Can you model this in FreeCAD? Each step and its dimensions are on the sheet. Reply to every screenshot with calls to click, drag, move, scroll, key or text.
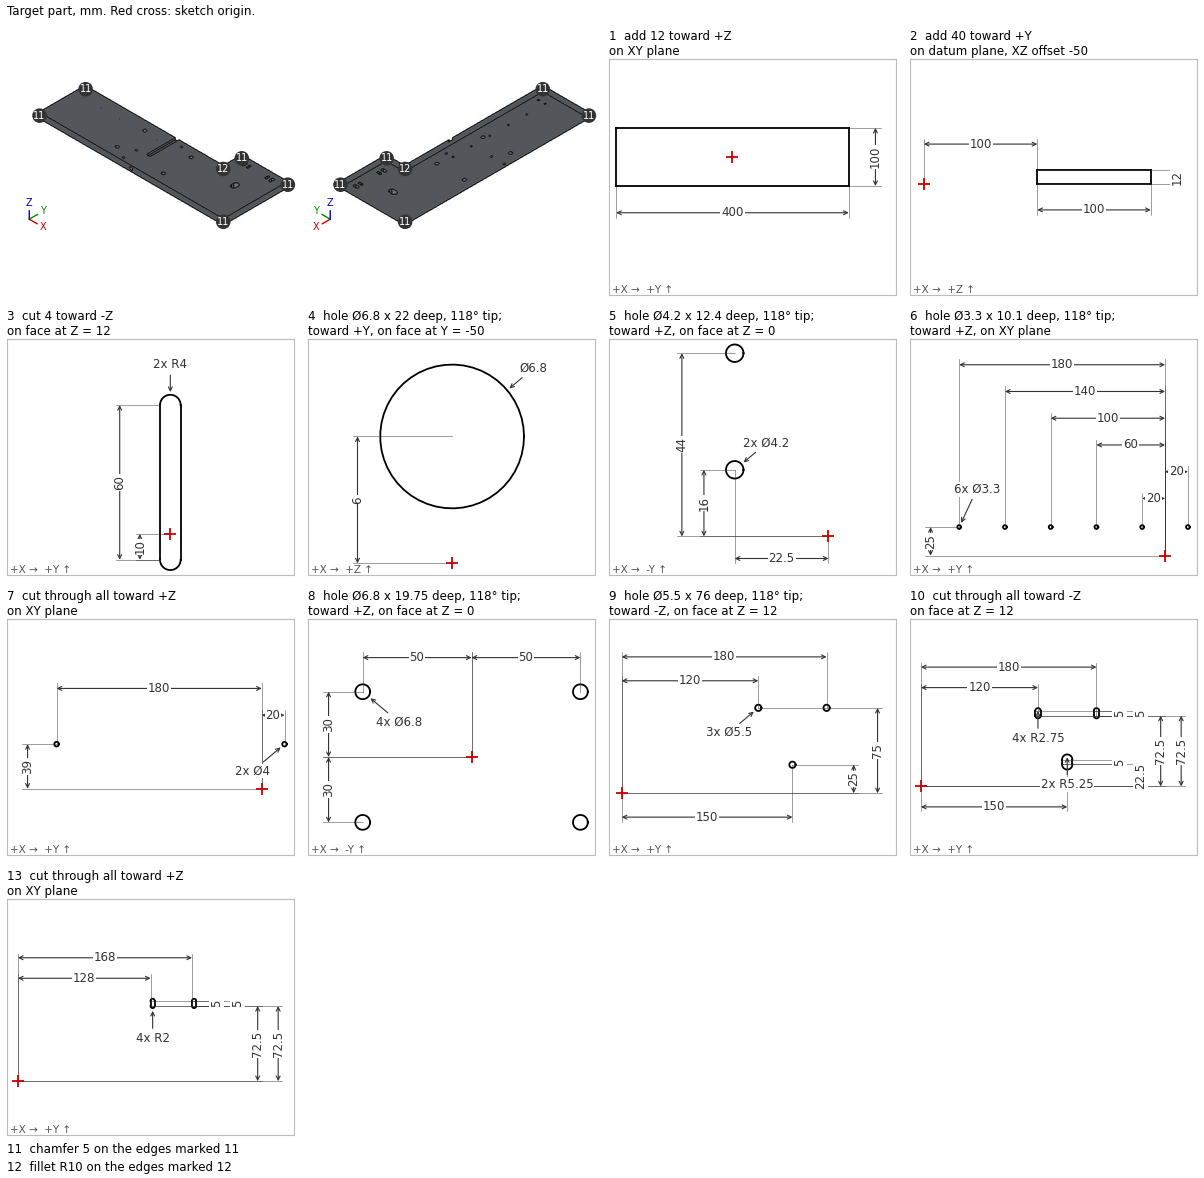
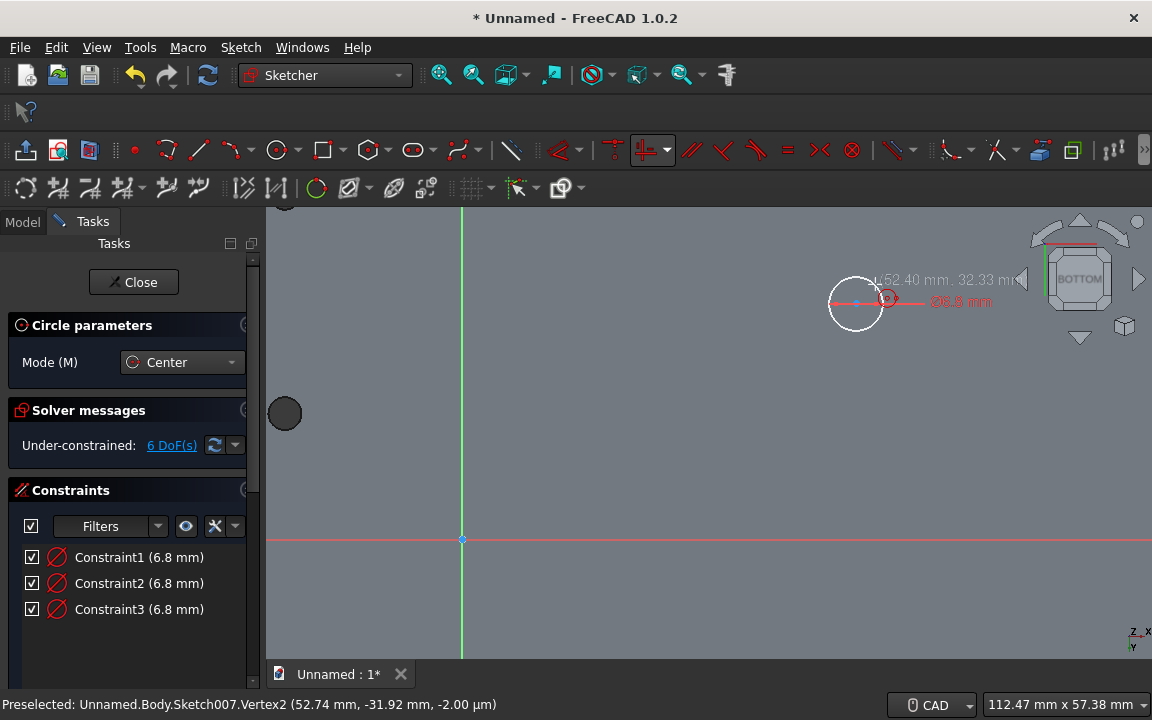
scroll(857, 303, down, 3)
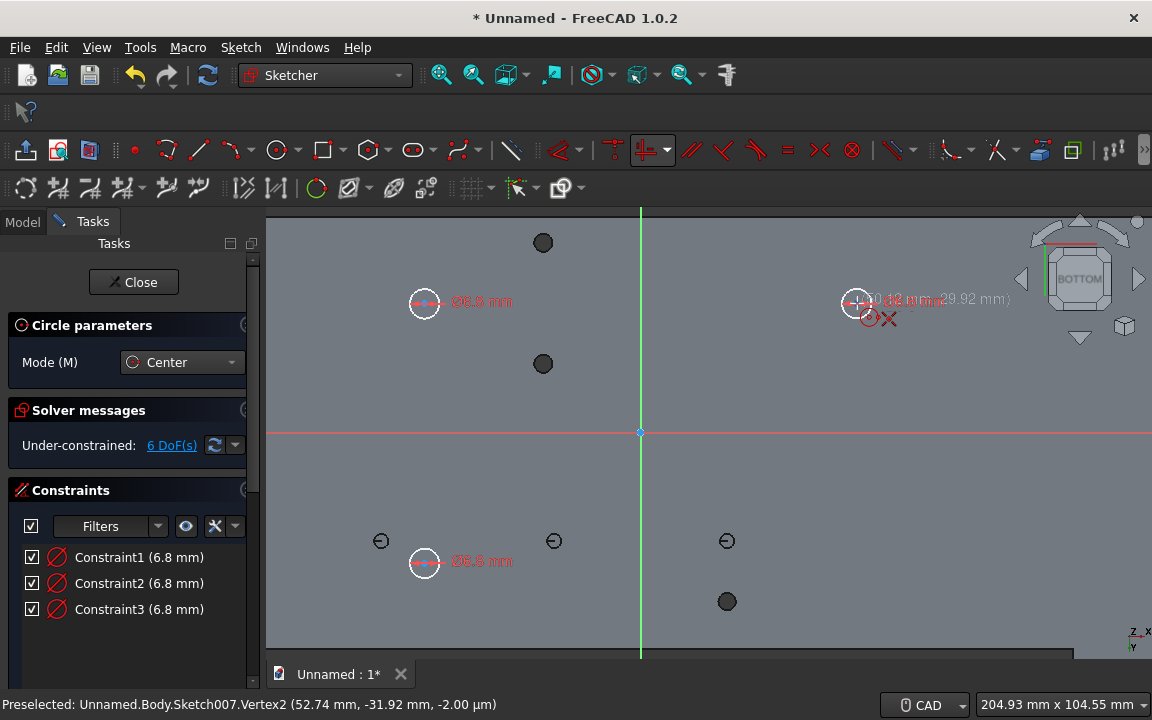
scroll(857, 563, up, 3)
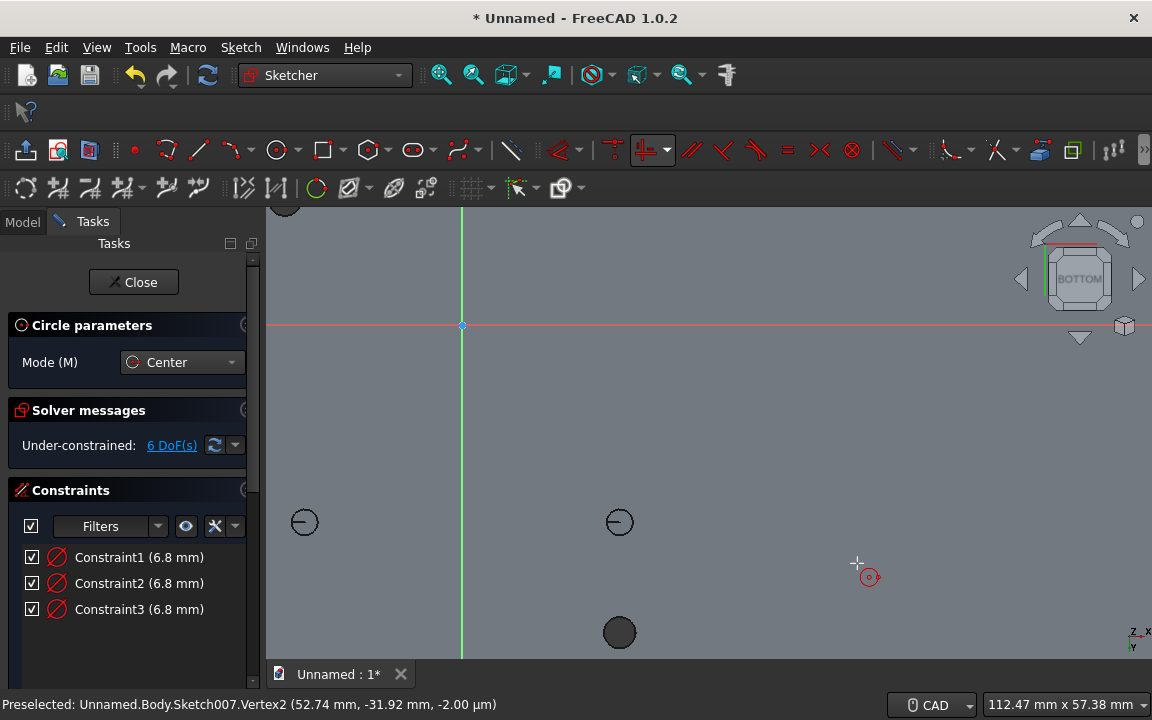
click(856, 562)
move(875, 543)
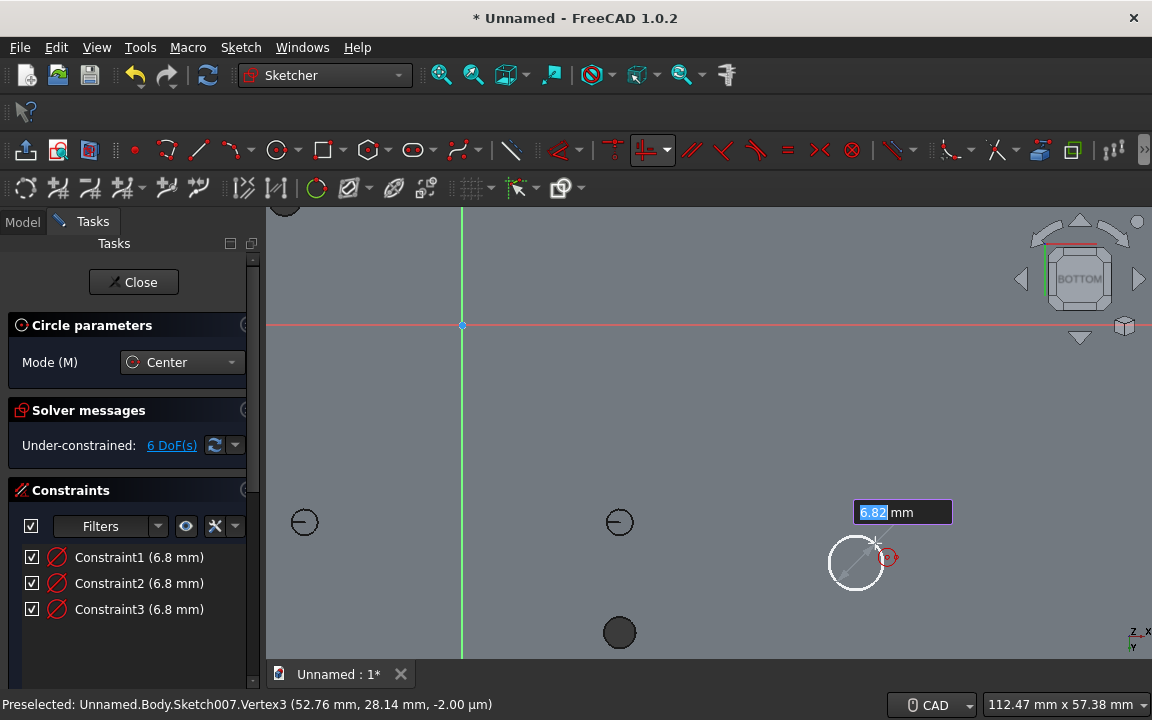
text(6.8)
key(Return)
key(Escape)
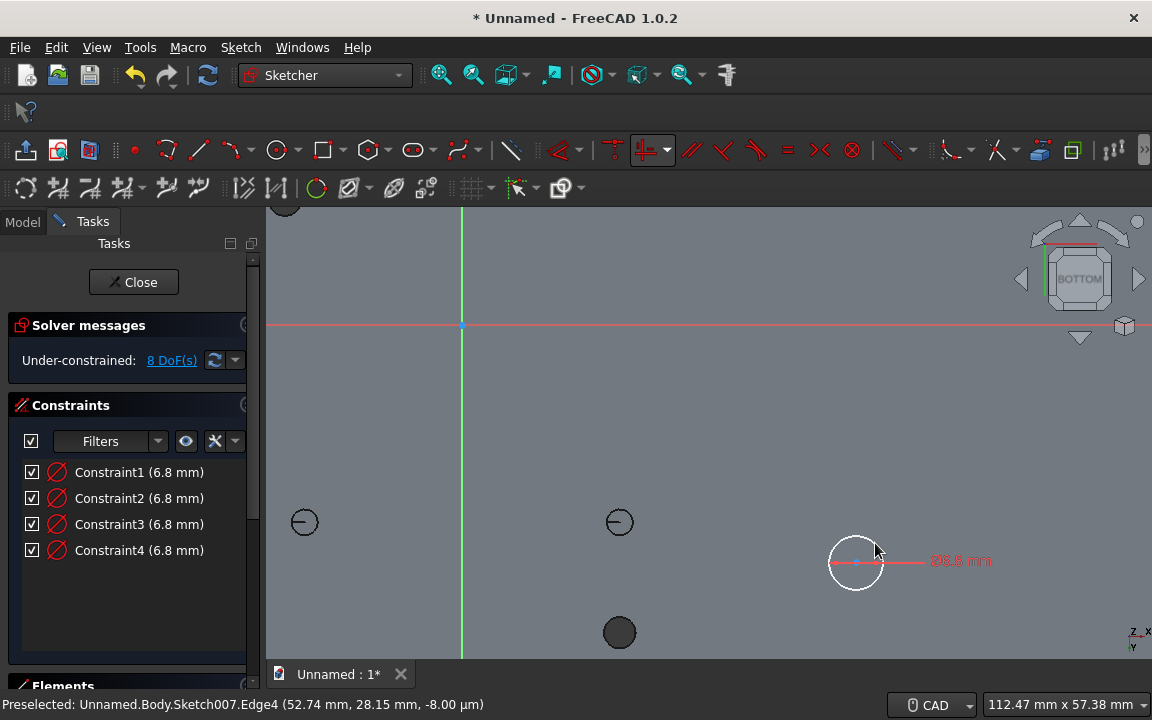
scroll(857, 564, down, 3)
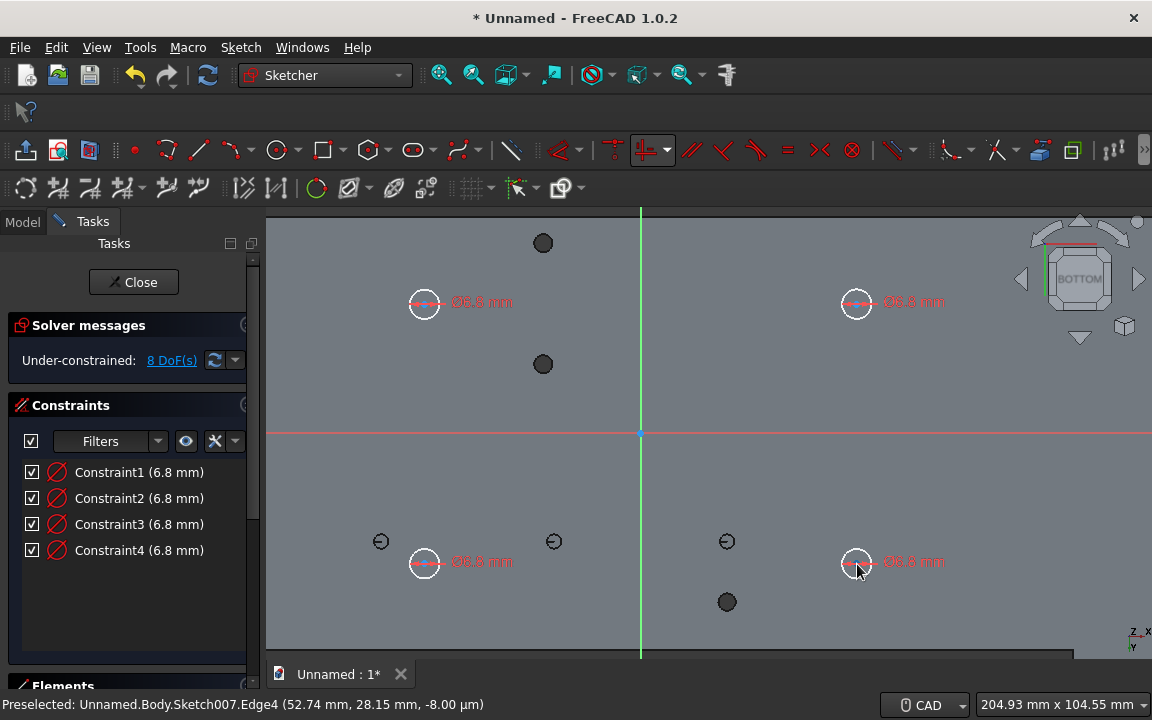
click(425, 304)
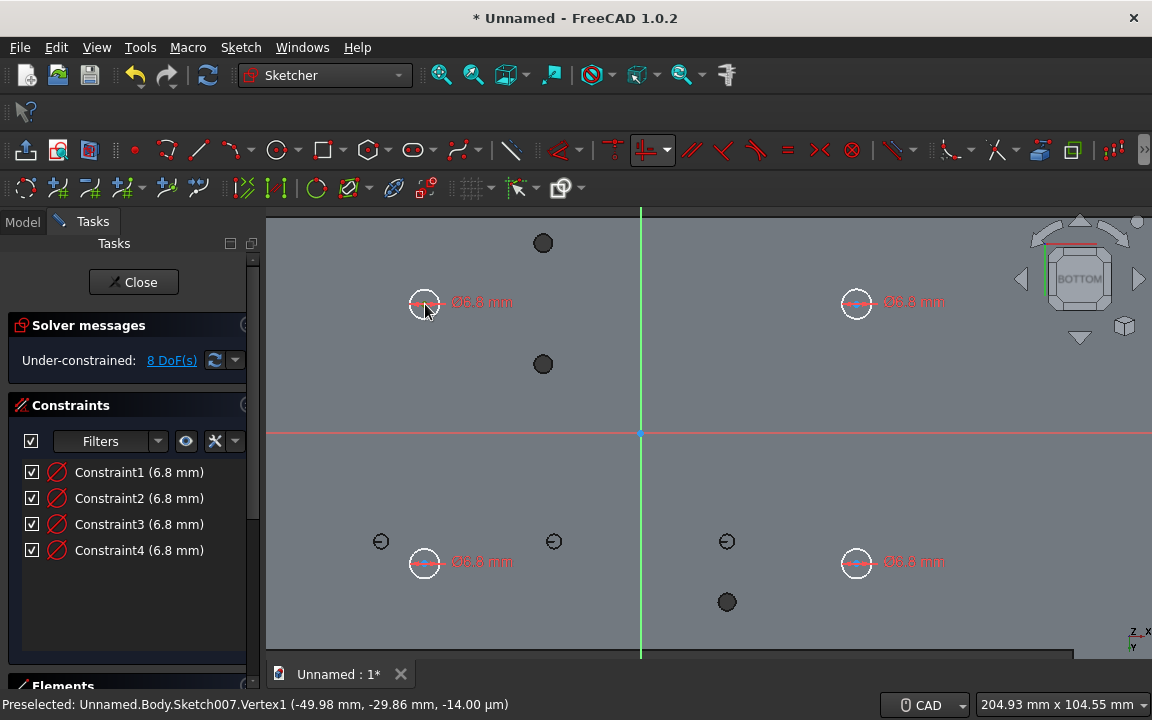
click(425, 564)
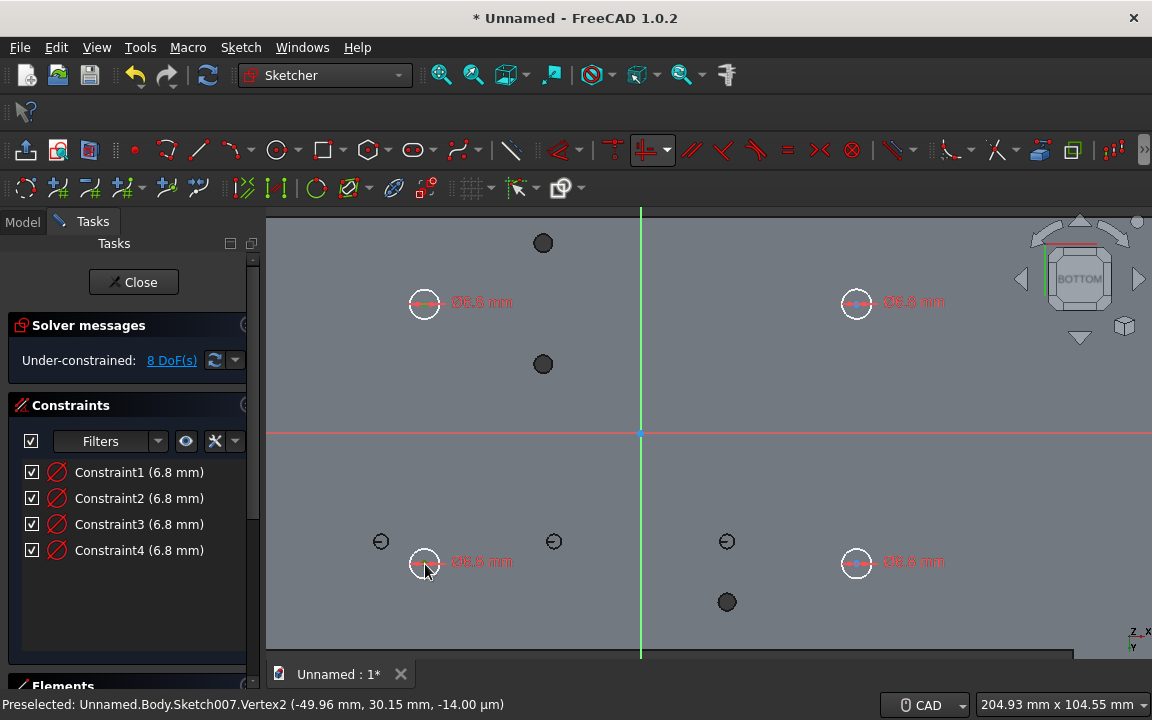
click(670, 150)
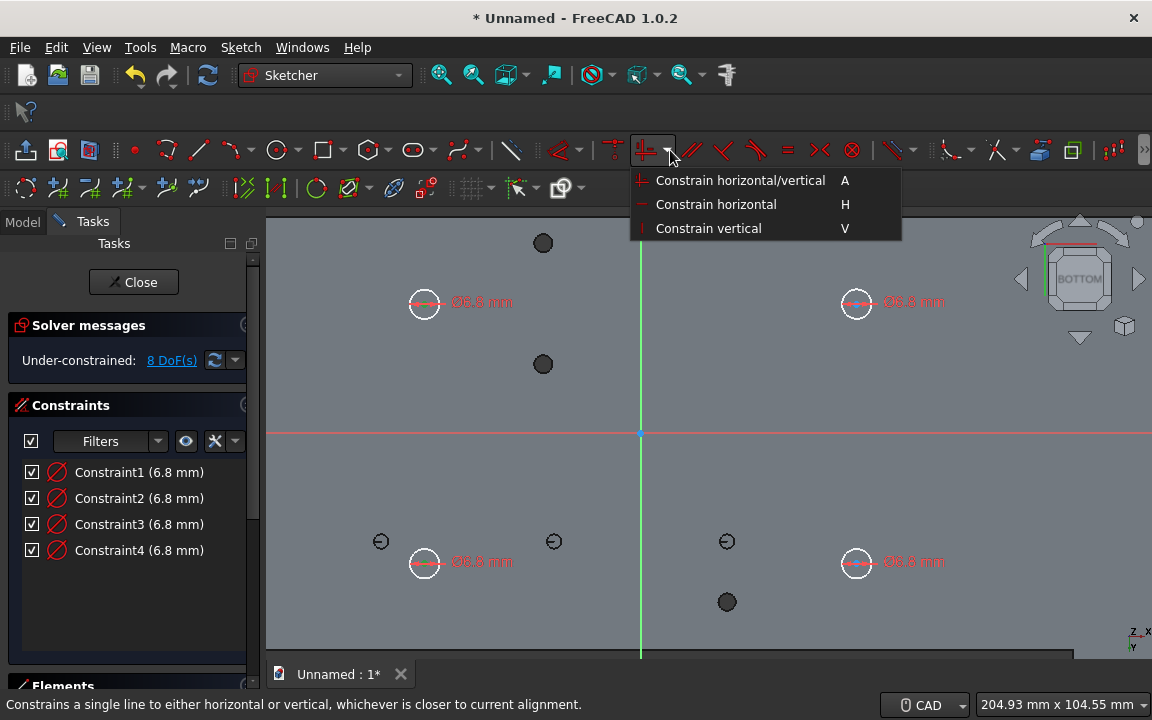
click(766, 228)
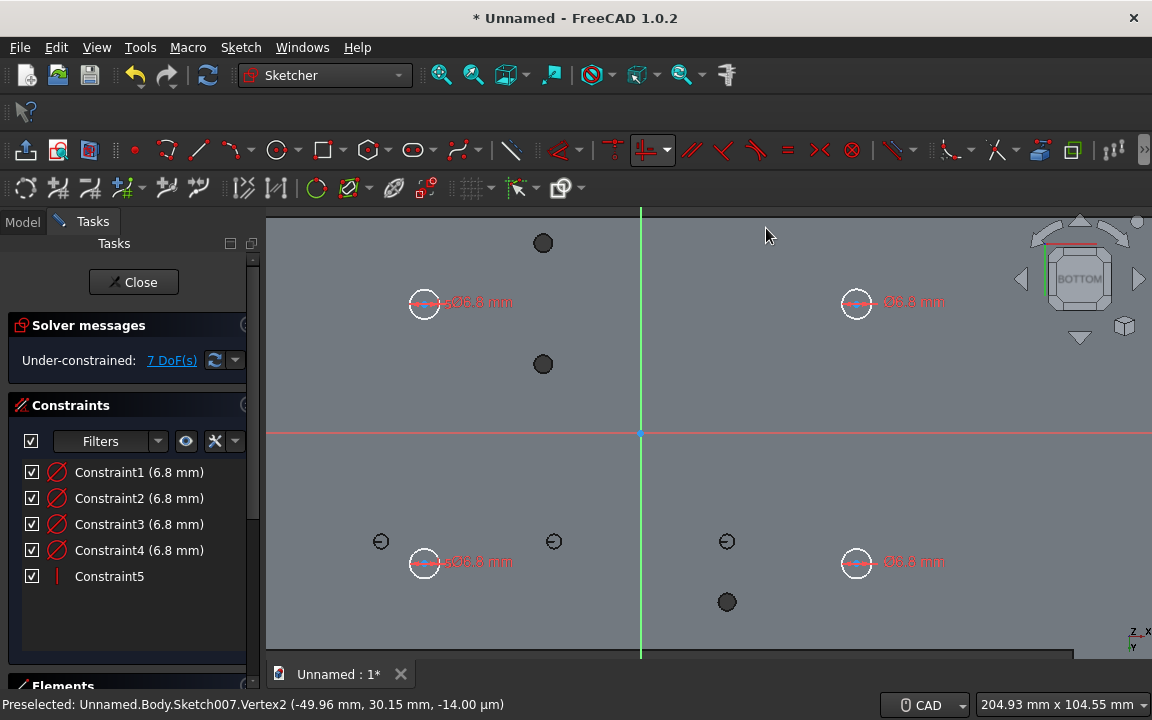
click(425, 304)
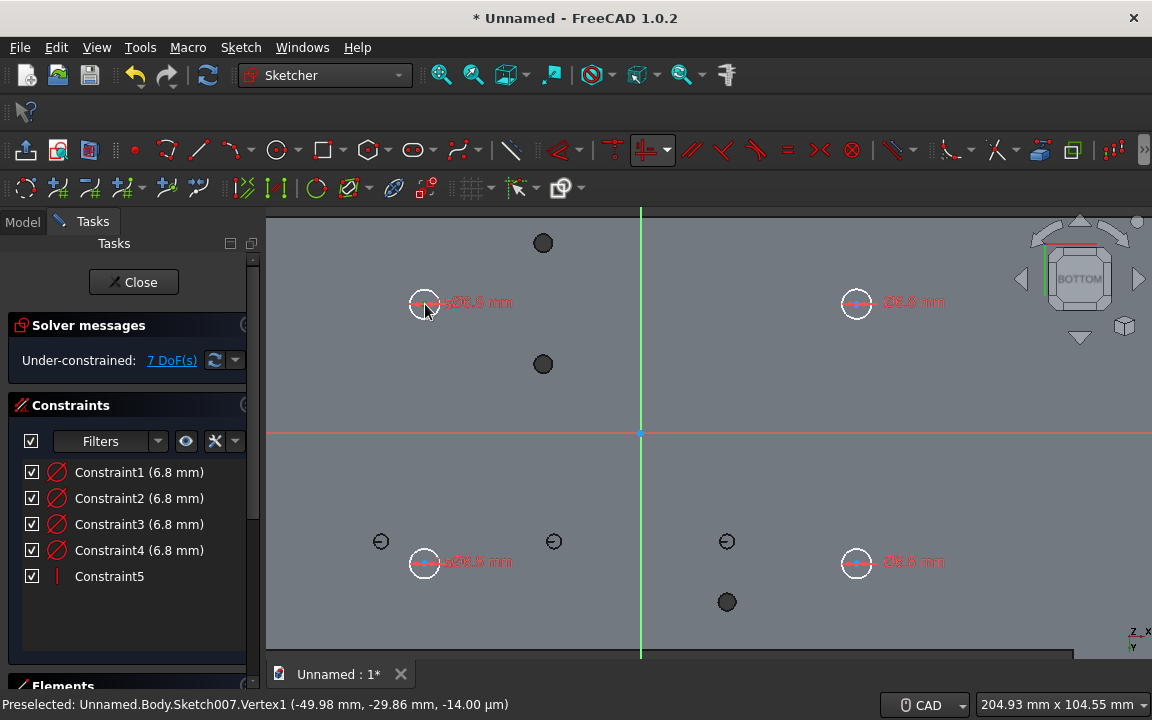
click(857, 304)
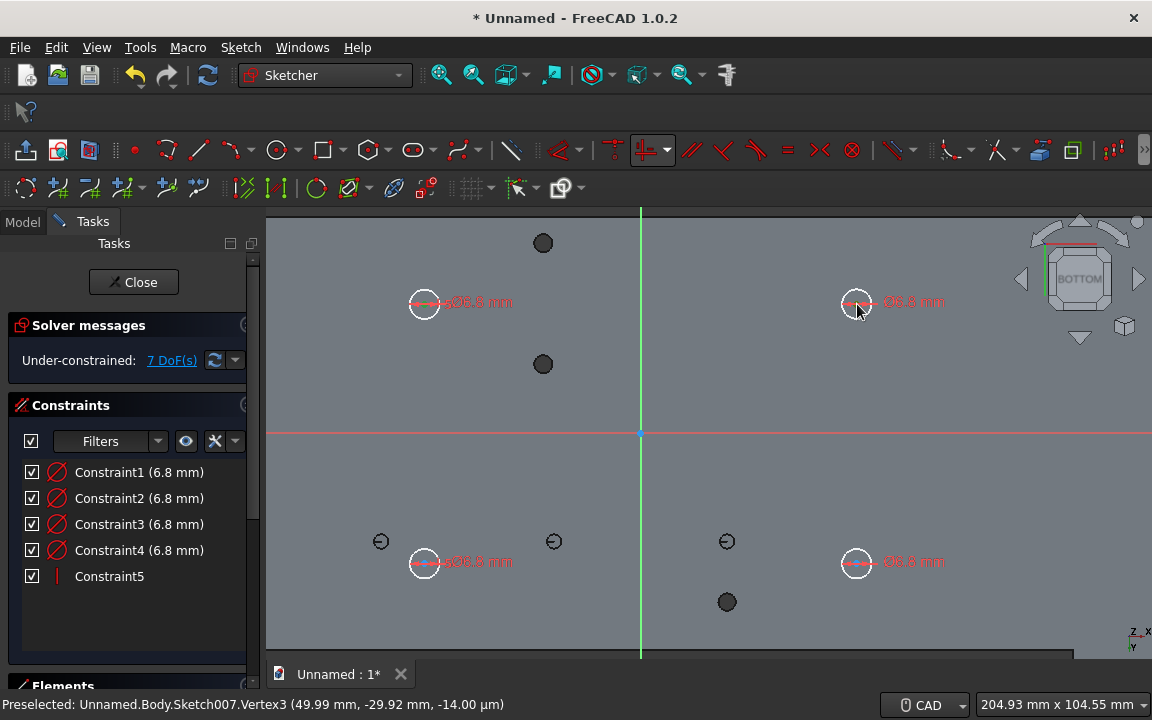
click(670, 150)